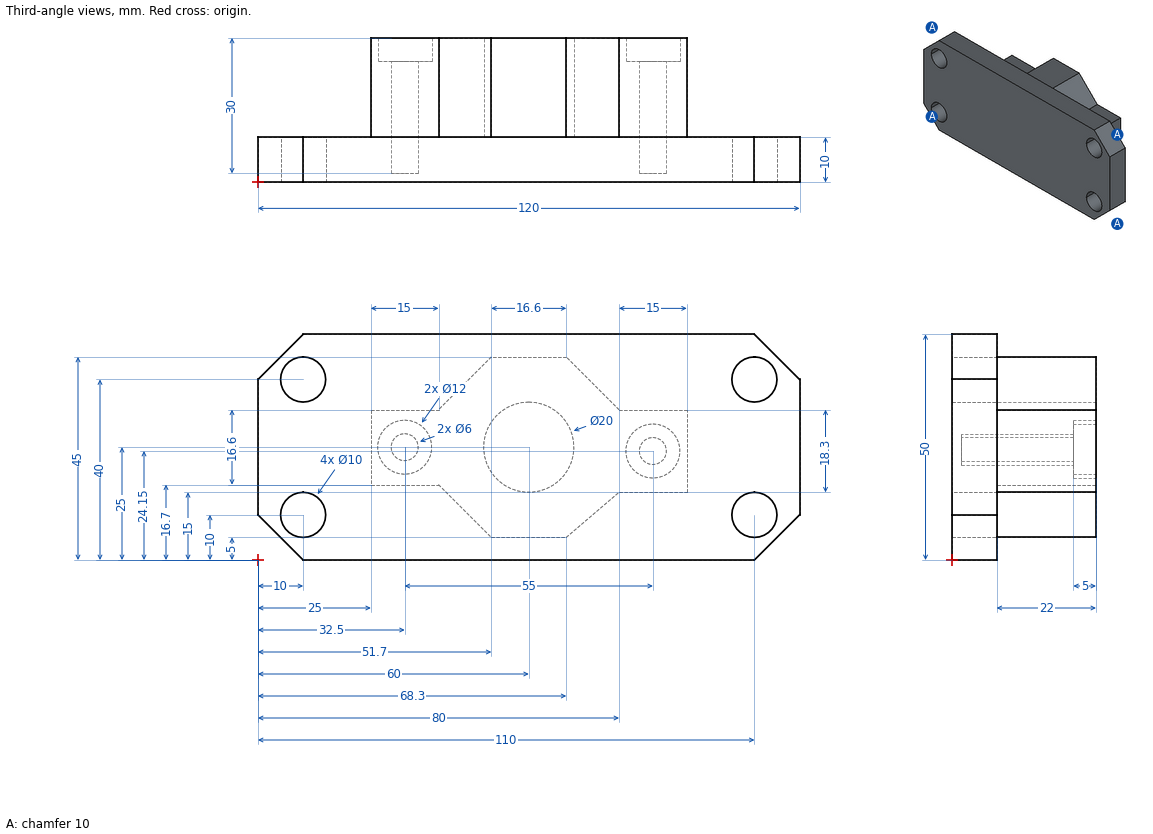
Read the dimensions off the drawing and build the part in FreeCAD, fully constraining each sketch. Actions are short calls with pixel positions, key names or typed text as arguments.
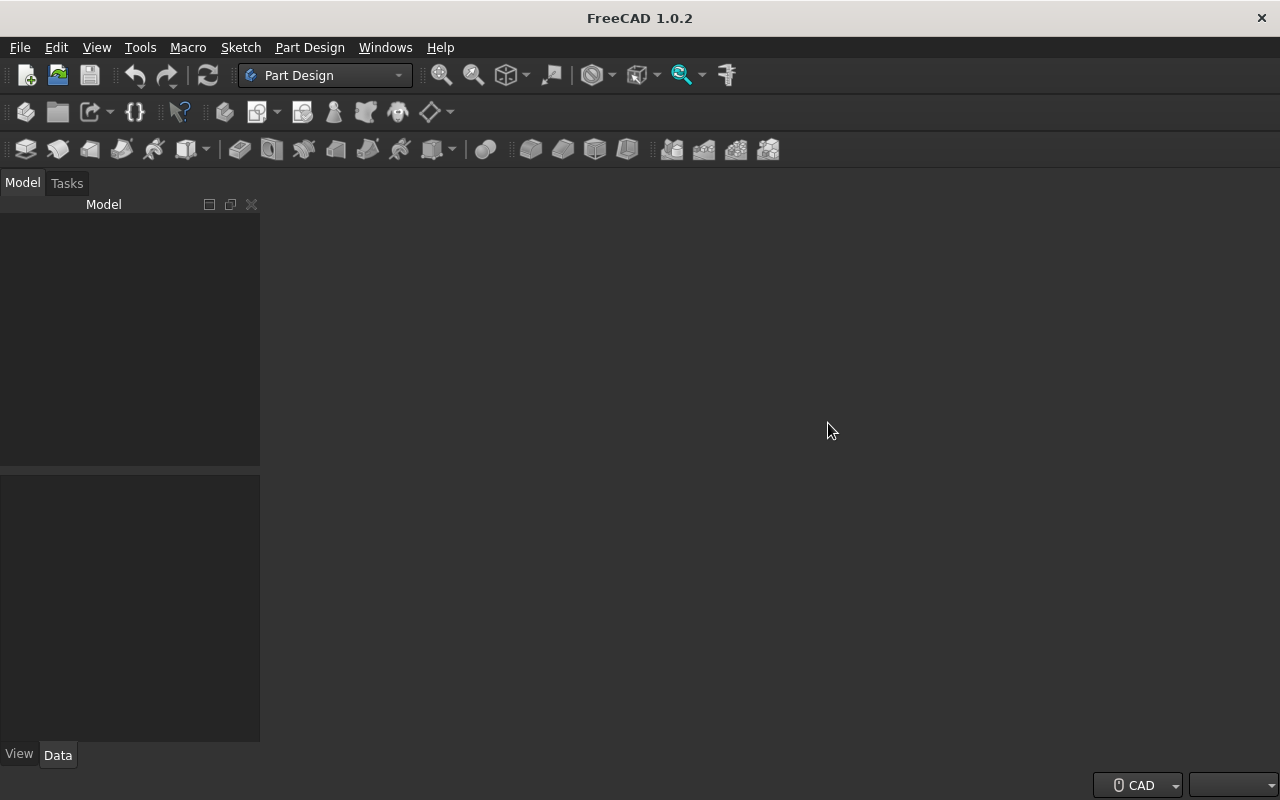
key(ctrl+n)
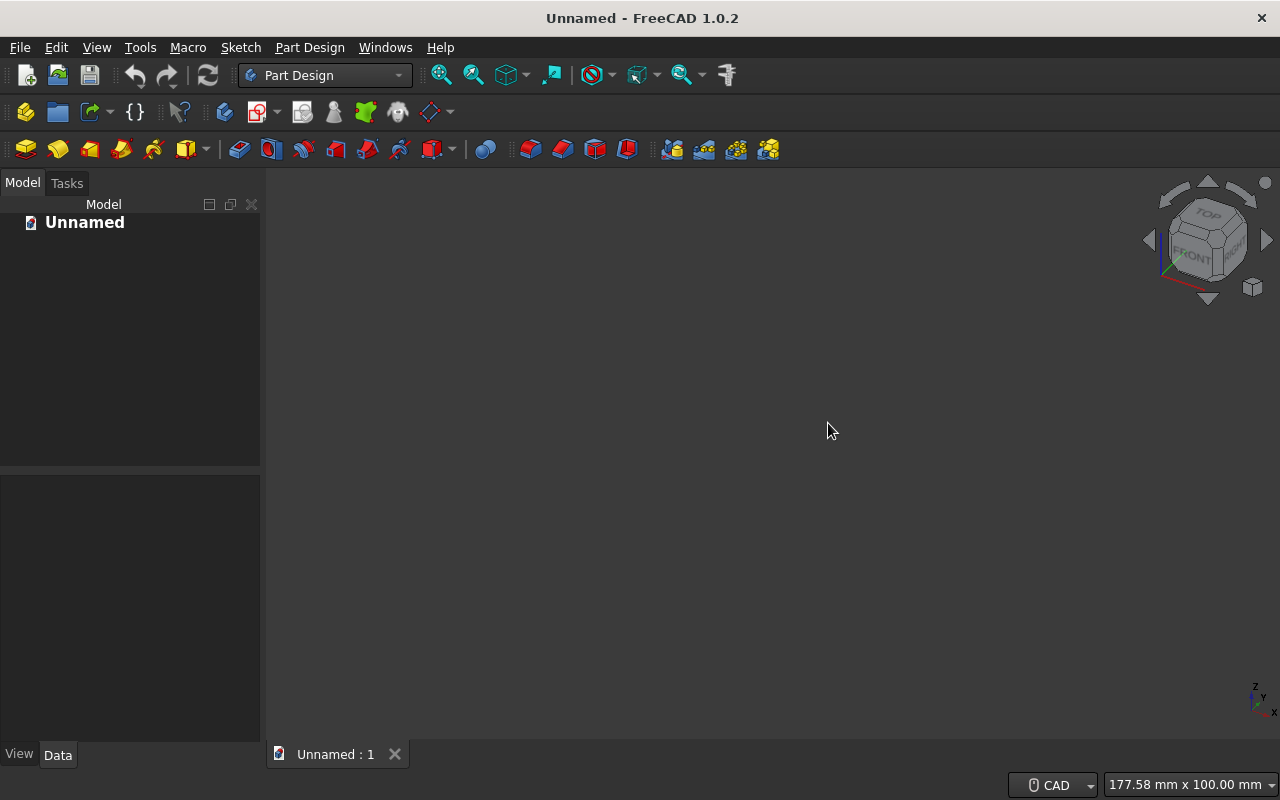
click(258, 112)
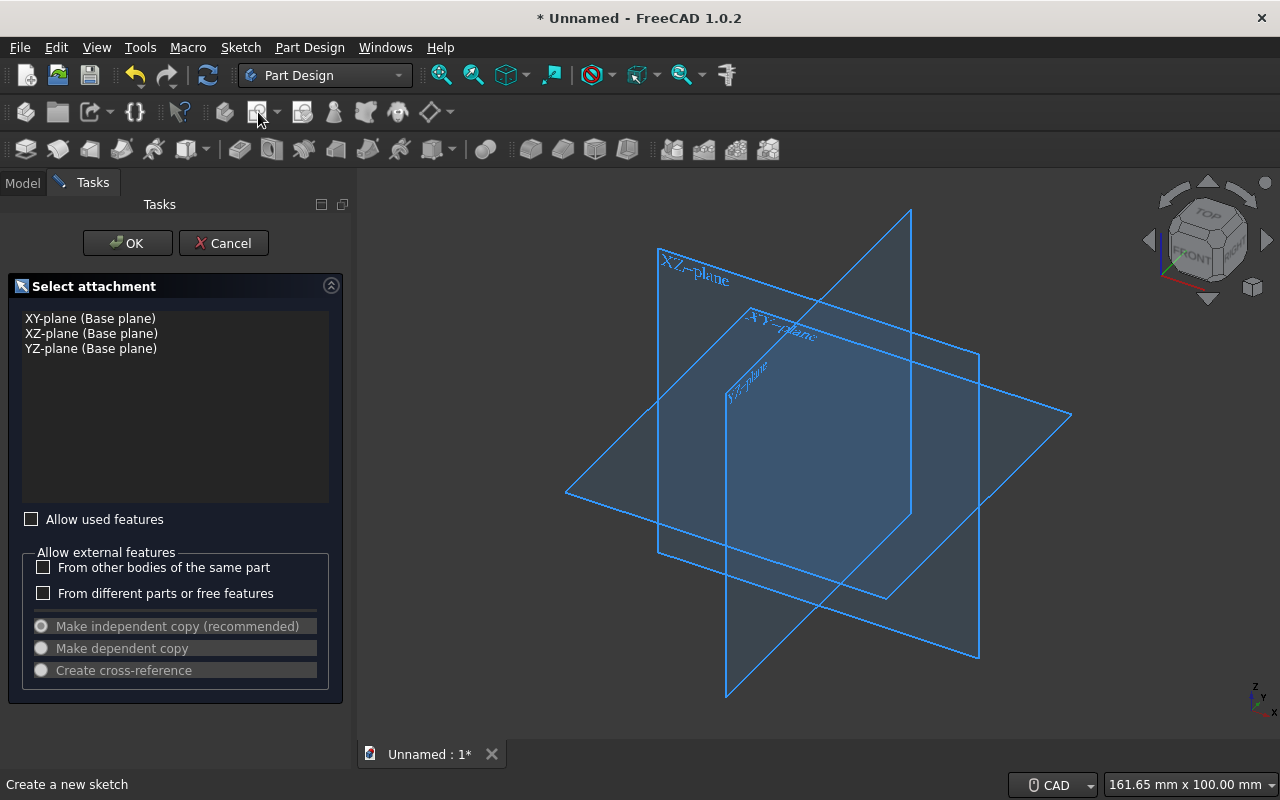
click(82, 318)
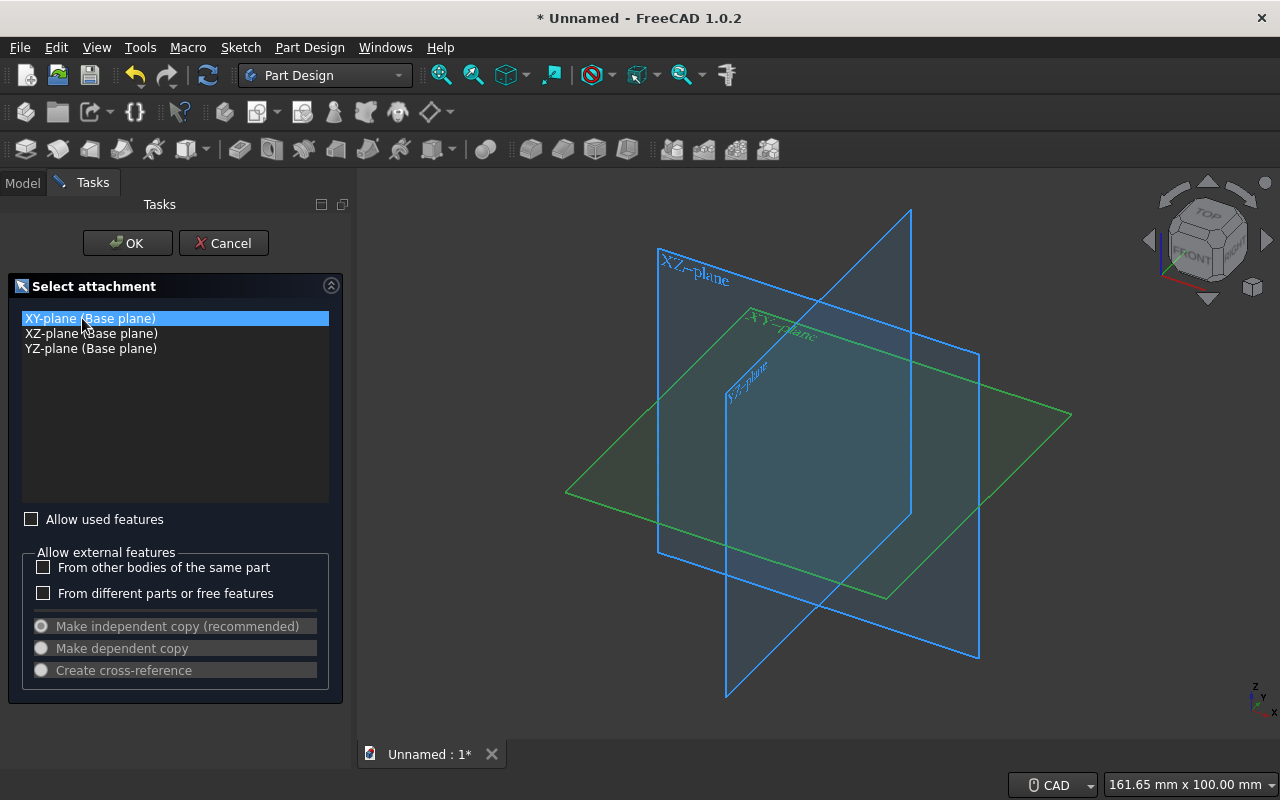
click(128, 243)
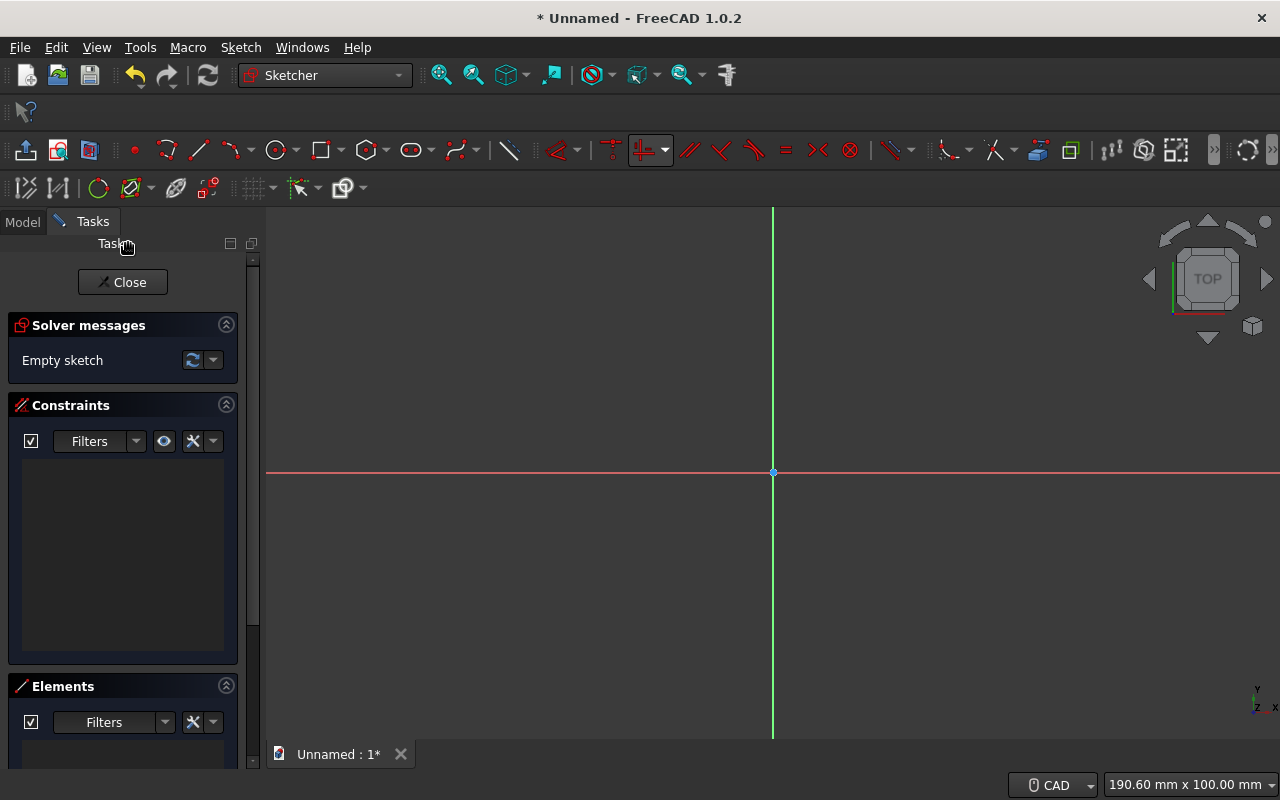
scroll(294, 527, down, 2)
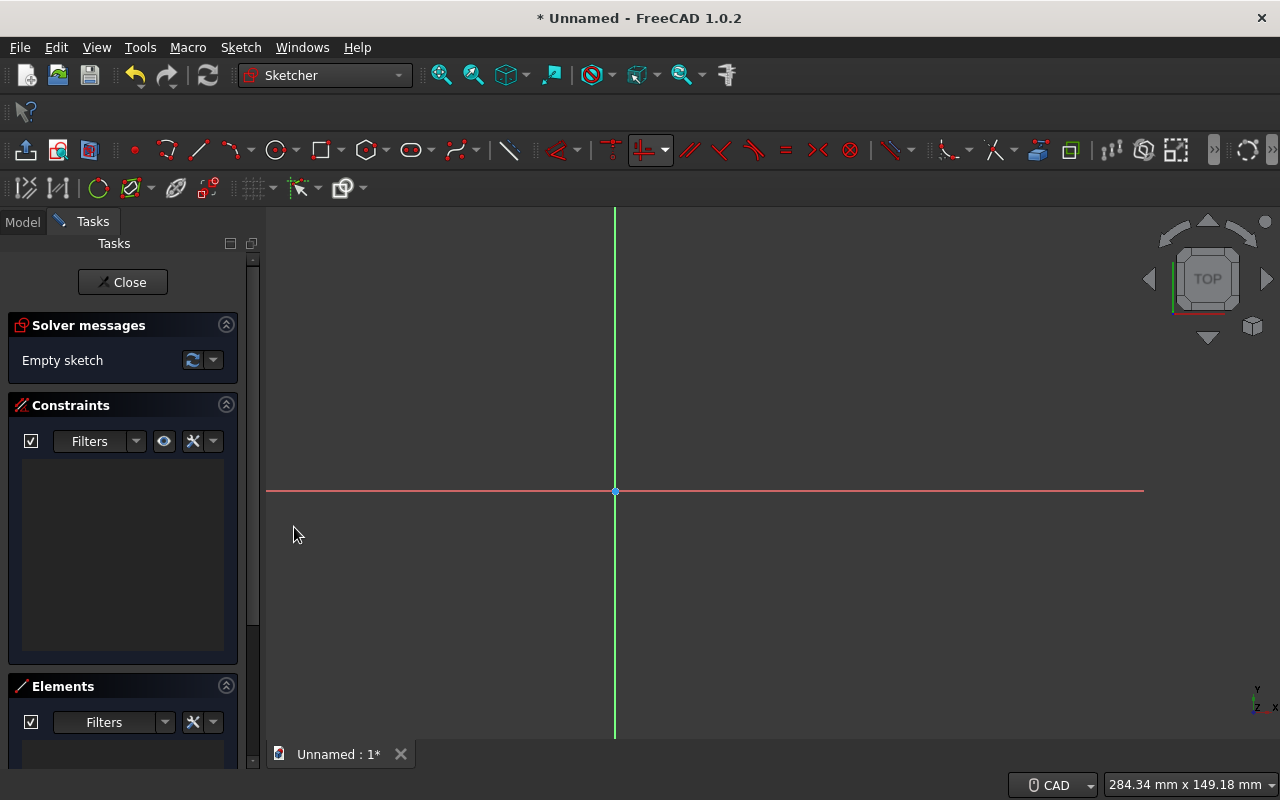
scroll(1082, 474, up, 2)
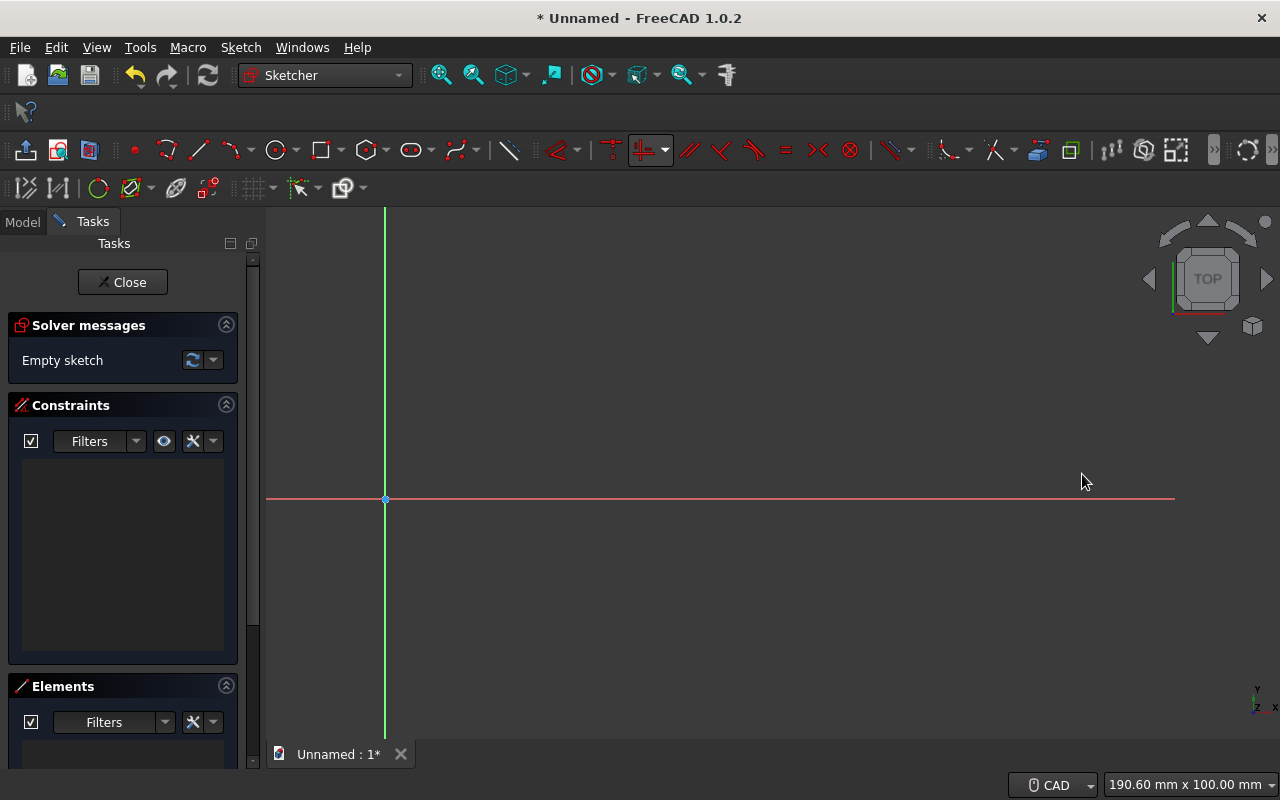
click(322, 150)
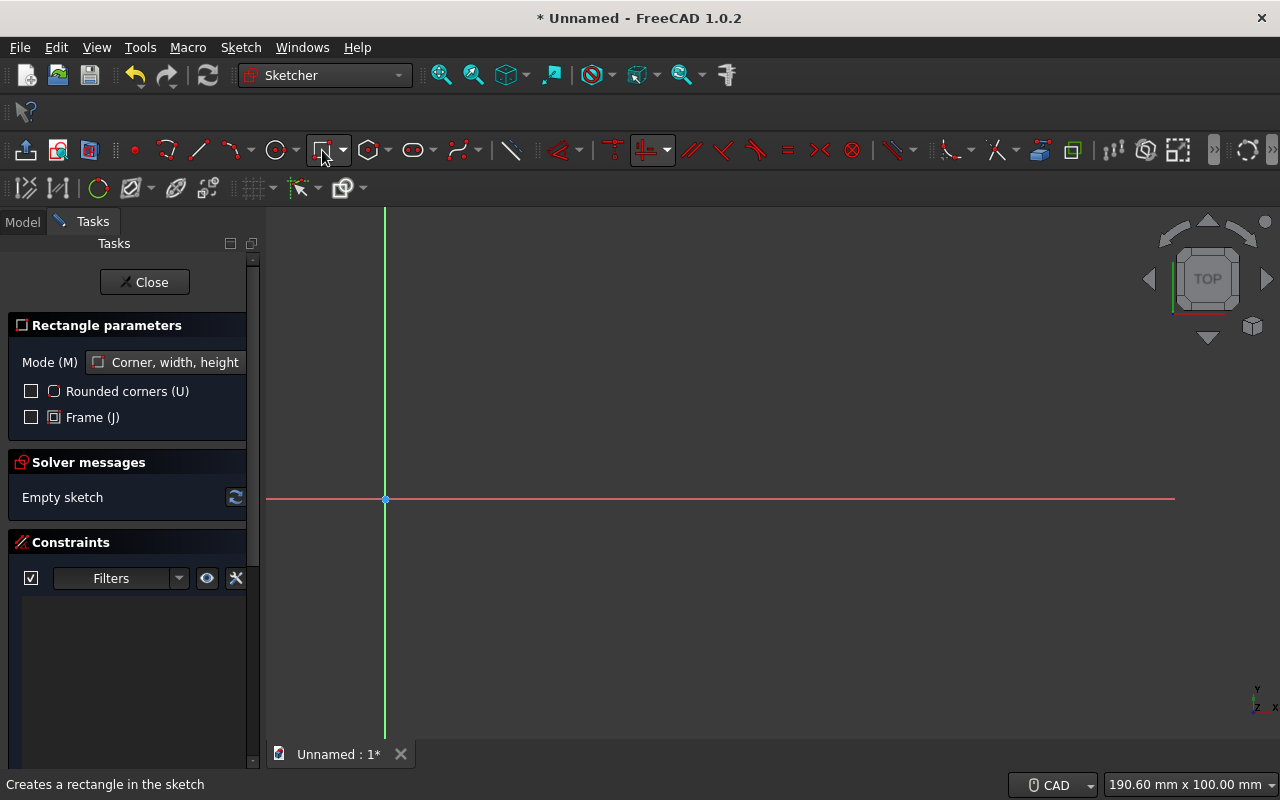
click(385, 499)
click(1023, 446)
key(Escape)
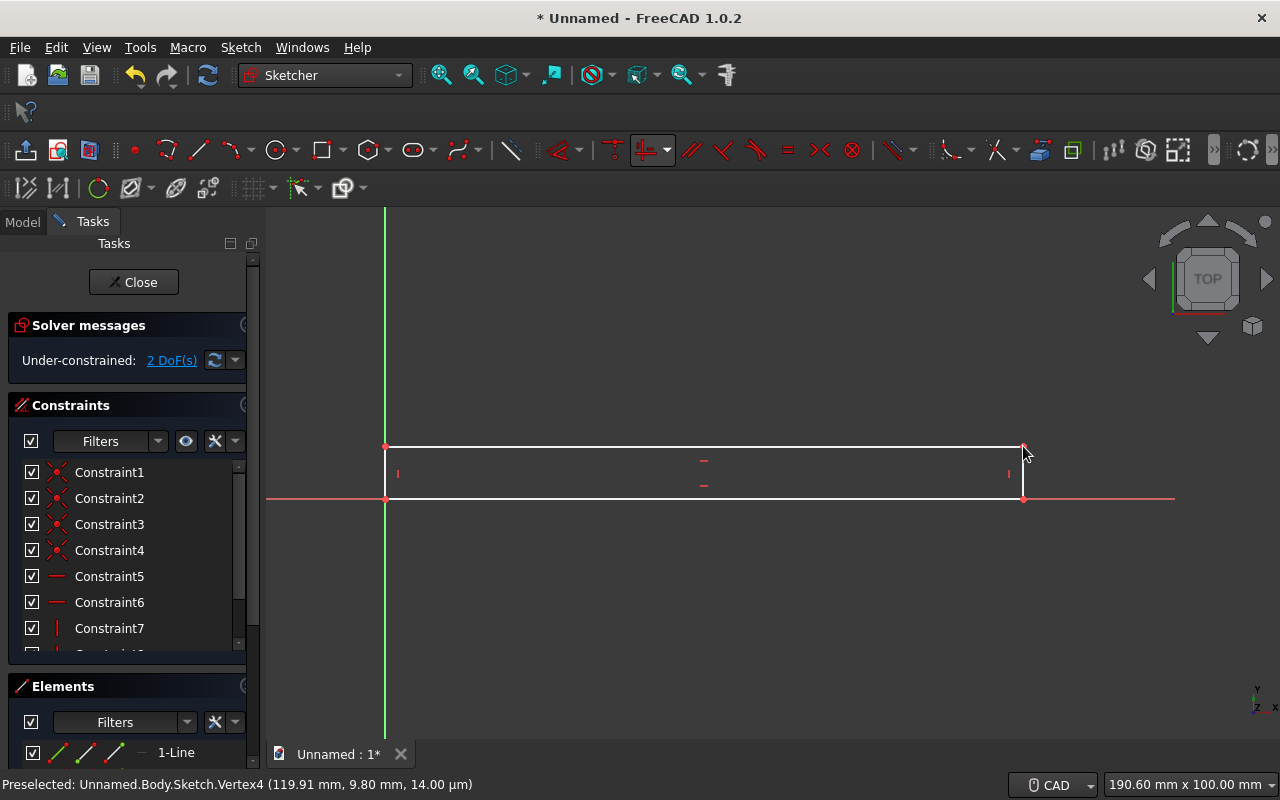
click(558, 150)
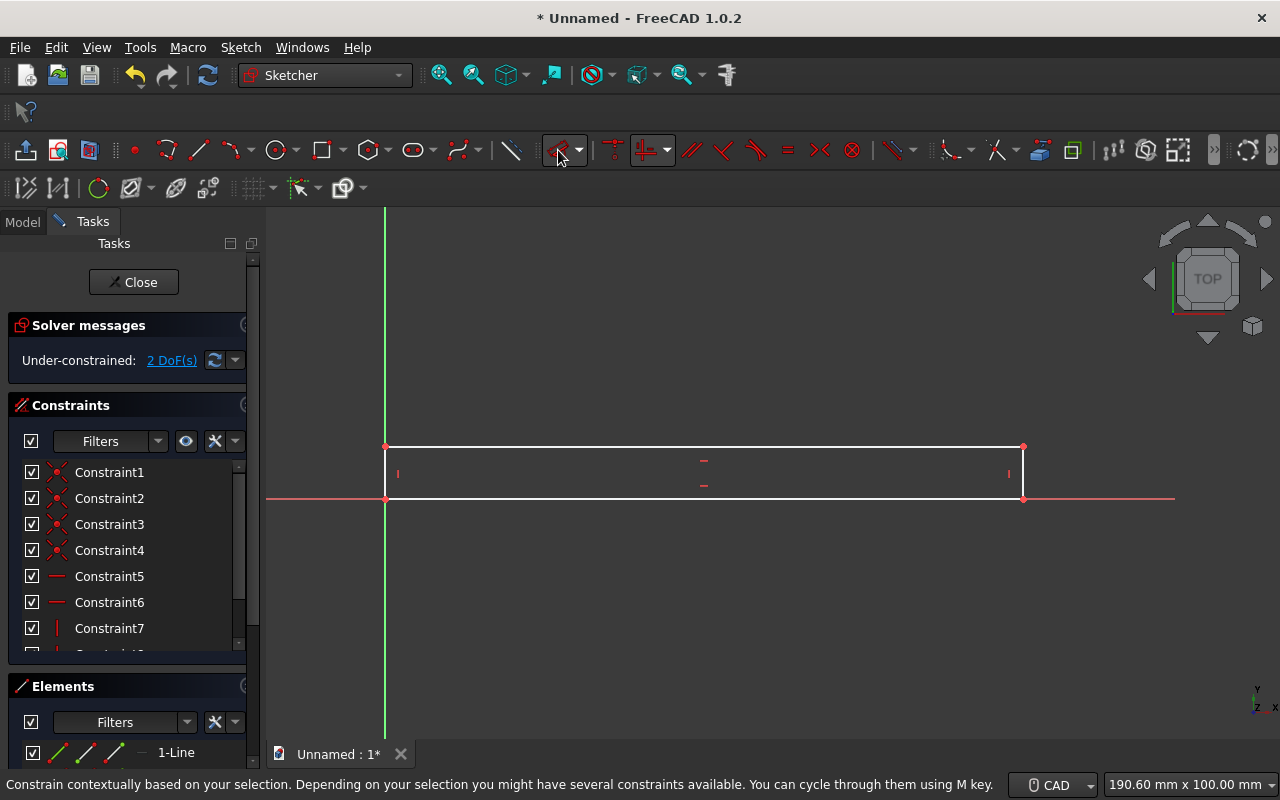
click(1023, 483)
click(1057, 473)